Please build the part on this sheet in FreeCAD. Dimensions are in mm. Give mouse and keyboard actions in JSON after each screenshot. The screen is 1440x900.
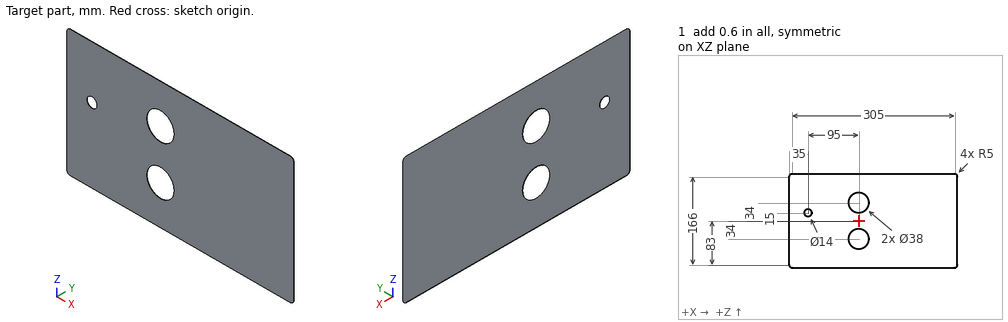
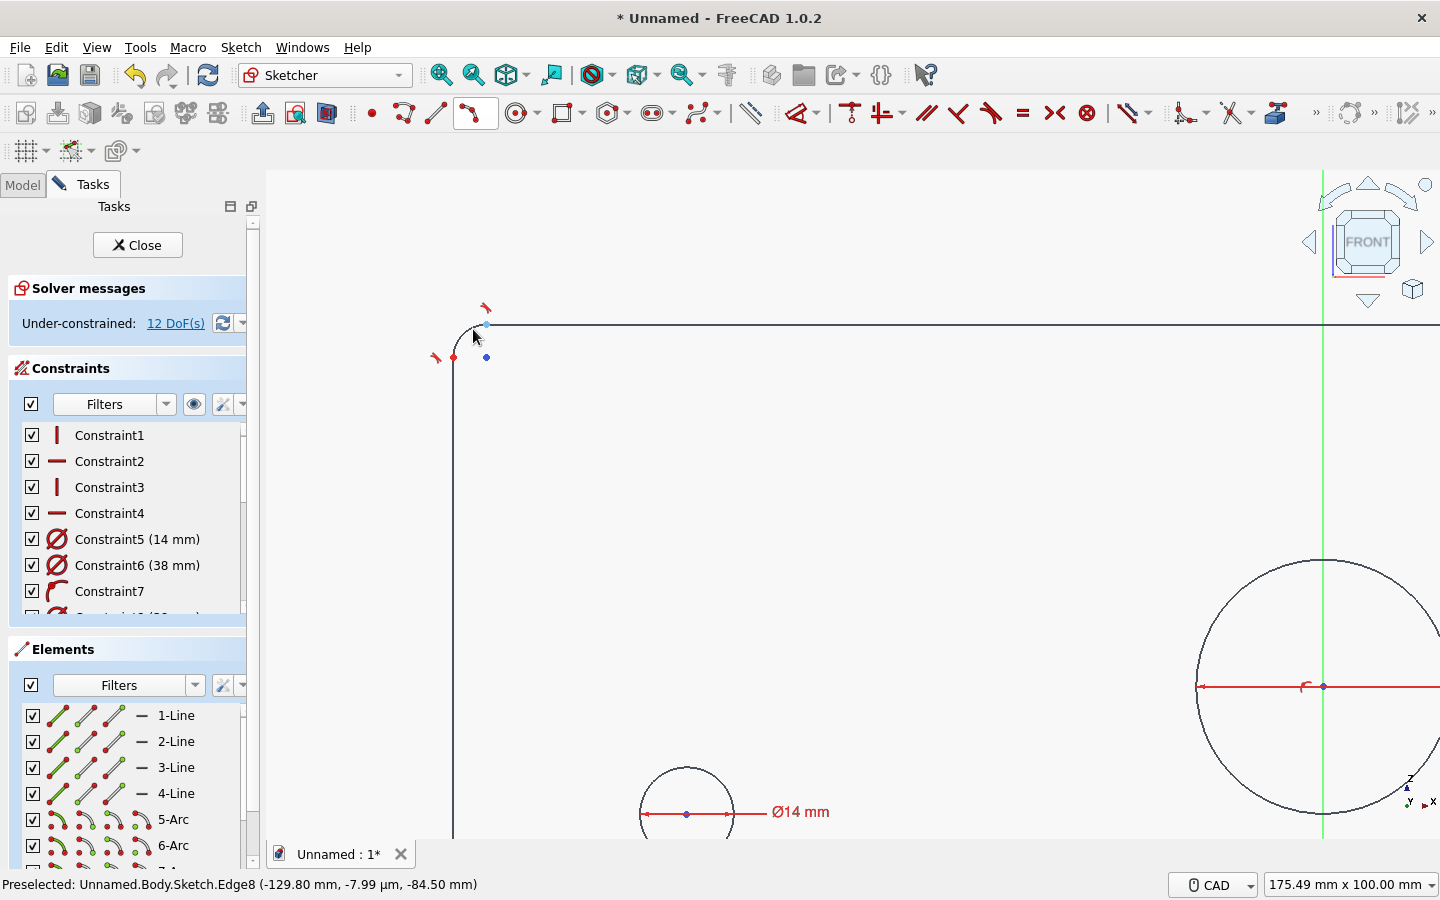
{"action": "left_click", "coordinate": [471, 328]}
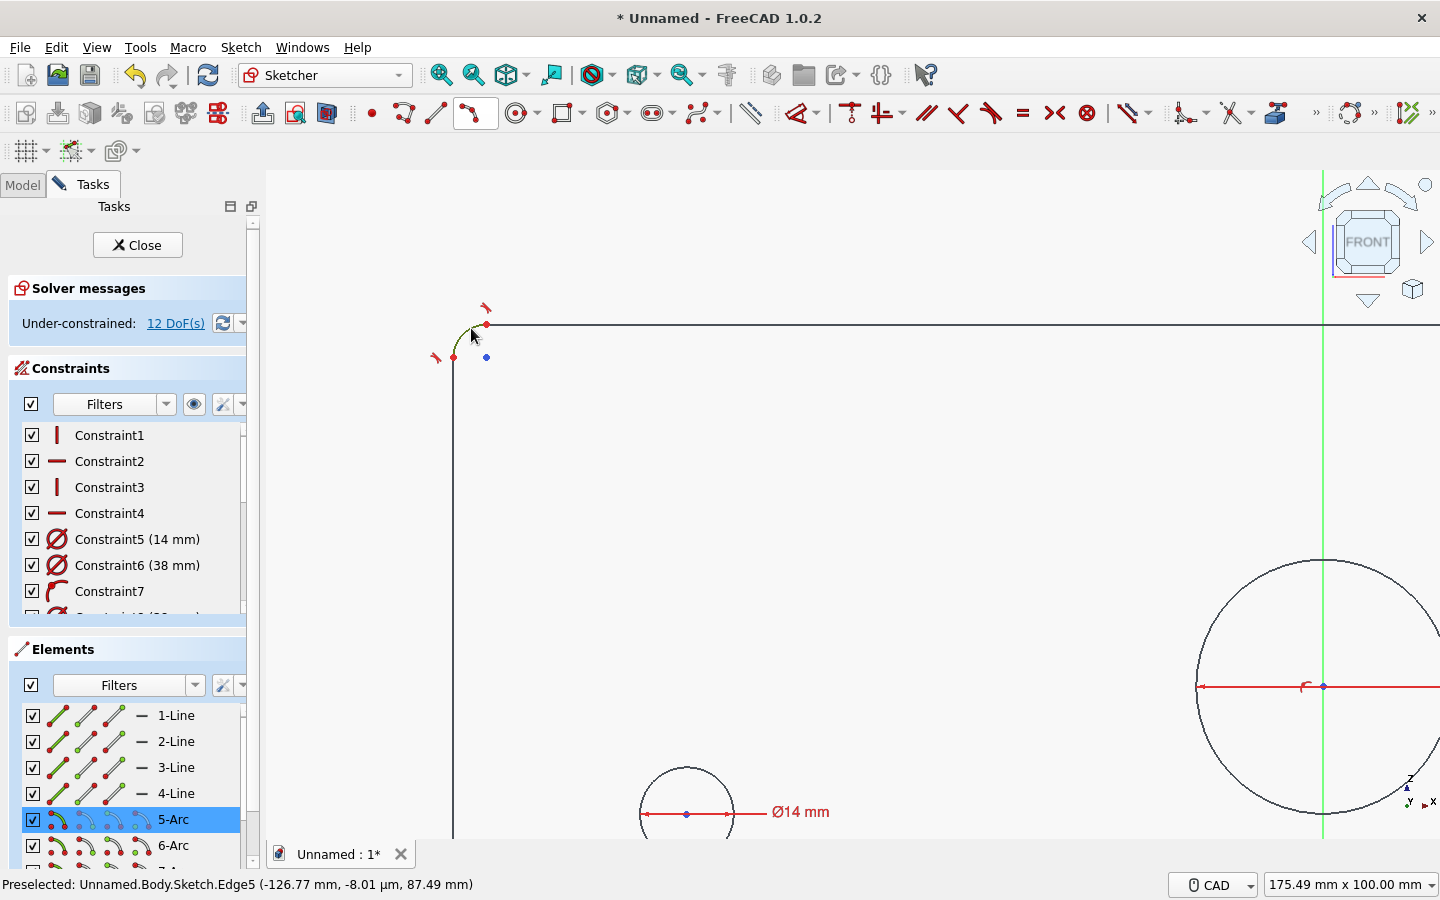
{"action": "scroll", "coordinate": [473, 329], "scroll_direction": "down", "scroll_amount": 6}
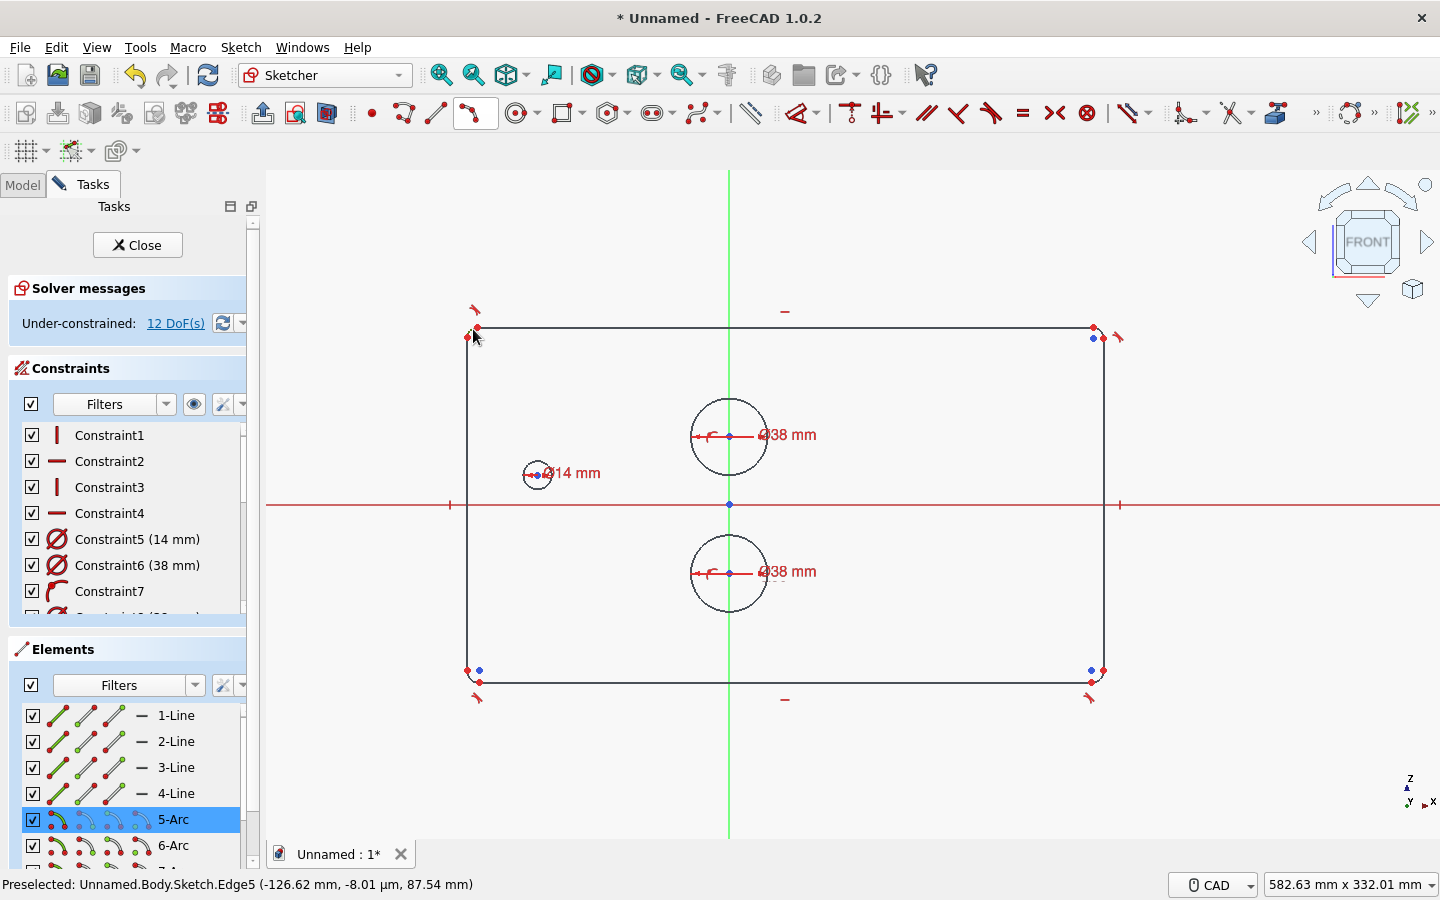
{"action": "scroll", "coordinate": [1102, 334], "scroll_direction": "up", "scroll_amount": 6}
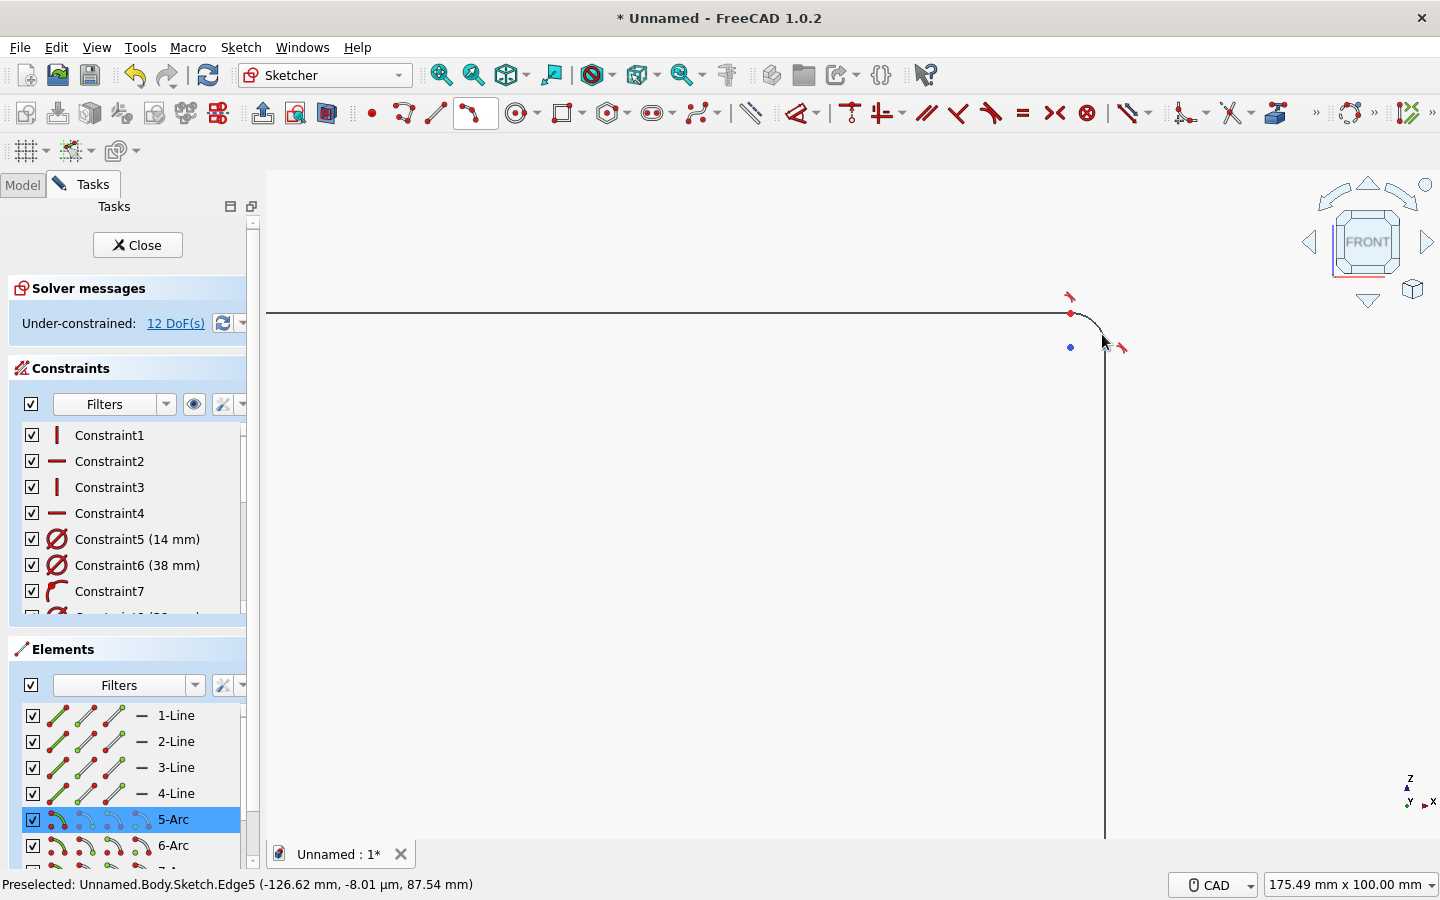
{"action": "left_click", "coordinate": [1102, 332]}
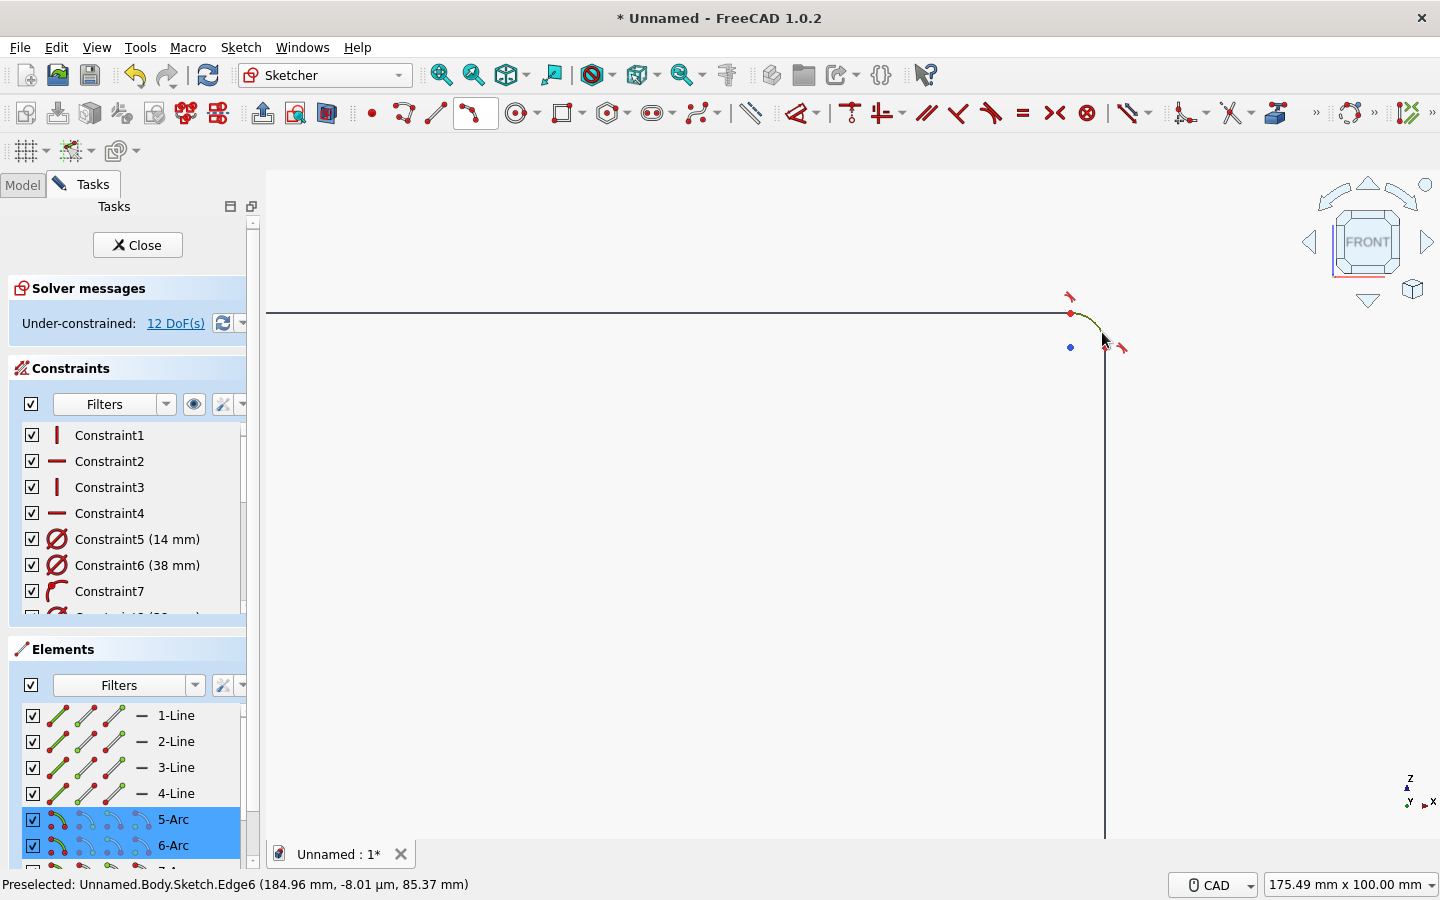
{"action": "scroll", "coordinate": [1103, 334], "scroll_direction": "down", "scroll_amount": 6}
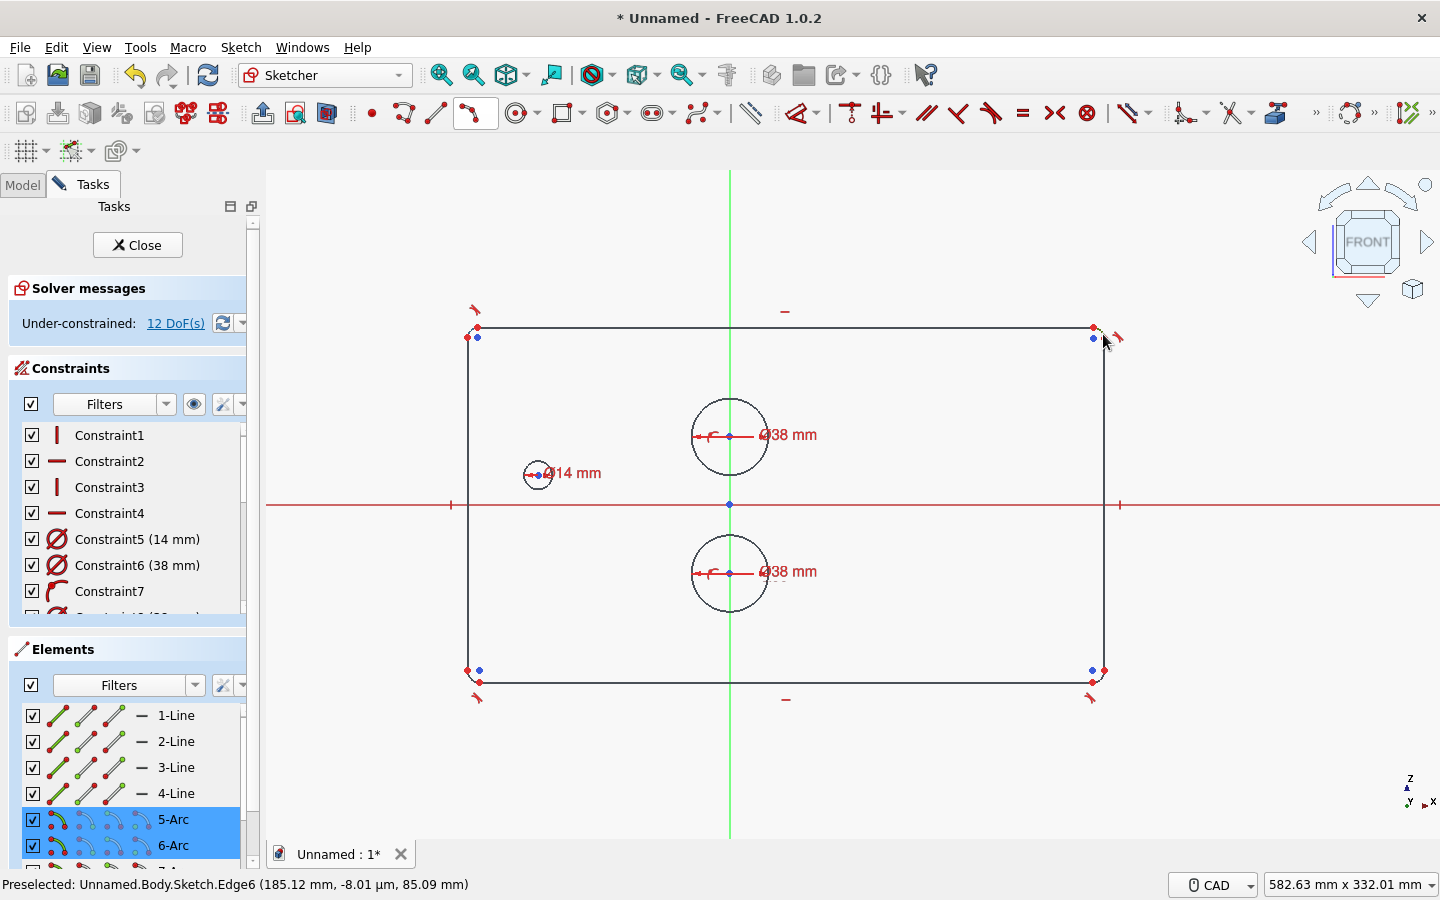
{"action": "scroll", "coordinate": [1098, 682], "scroll_direction": "up", "scroll_amount": 5}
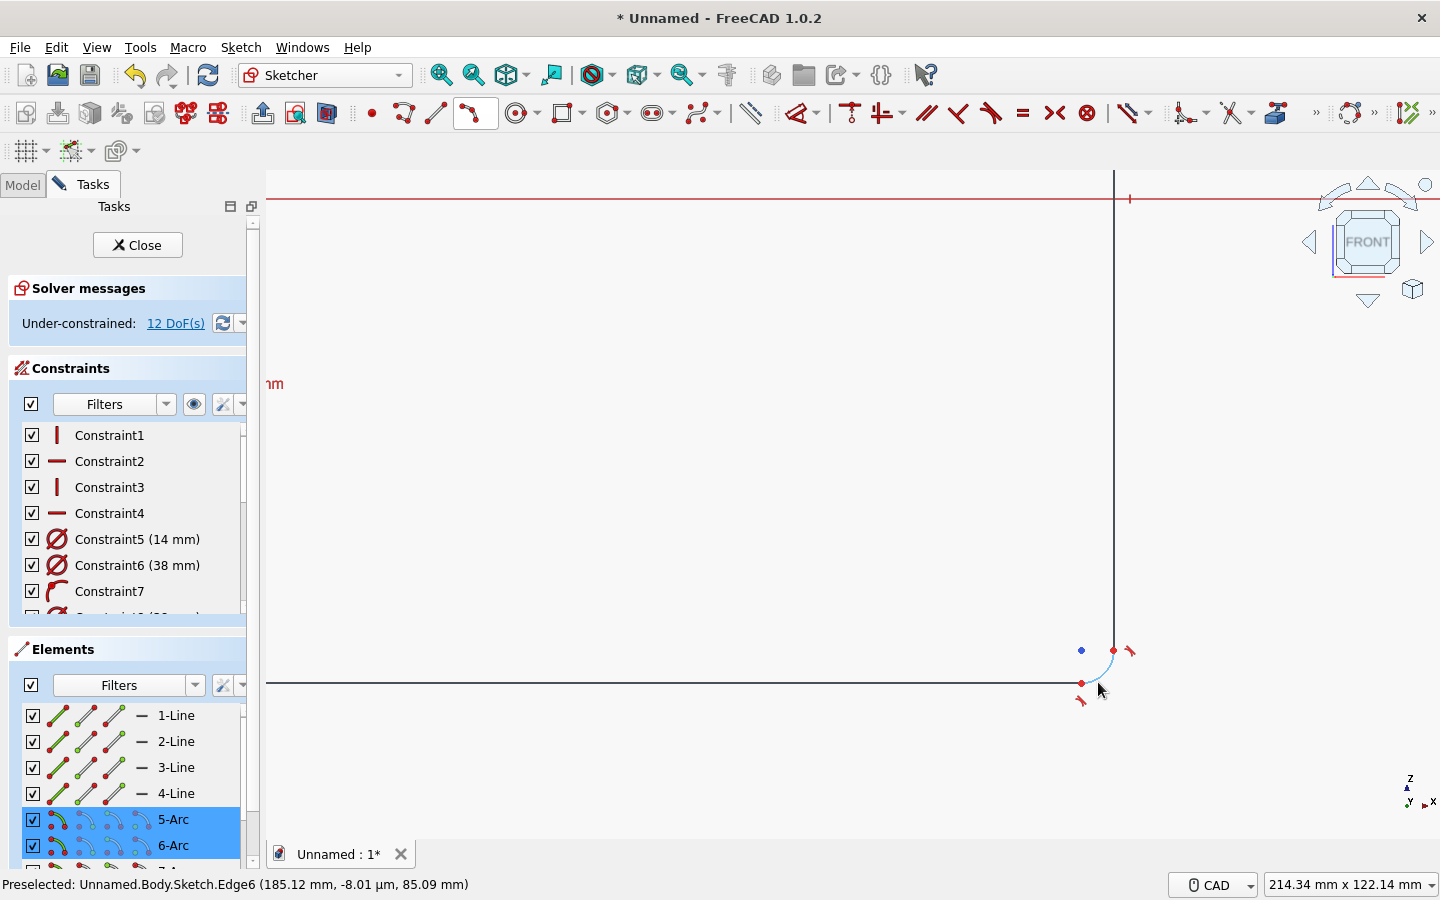
{"action": "left_click", "coordinate": [1096, 680]}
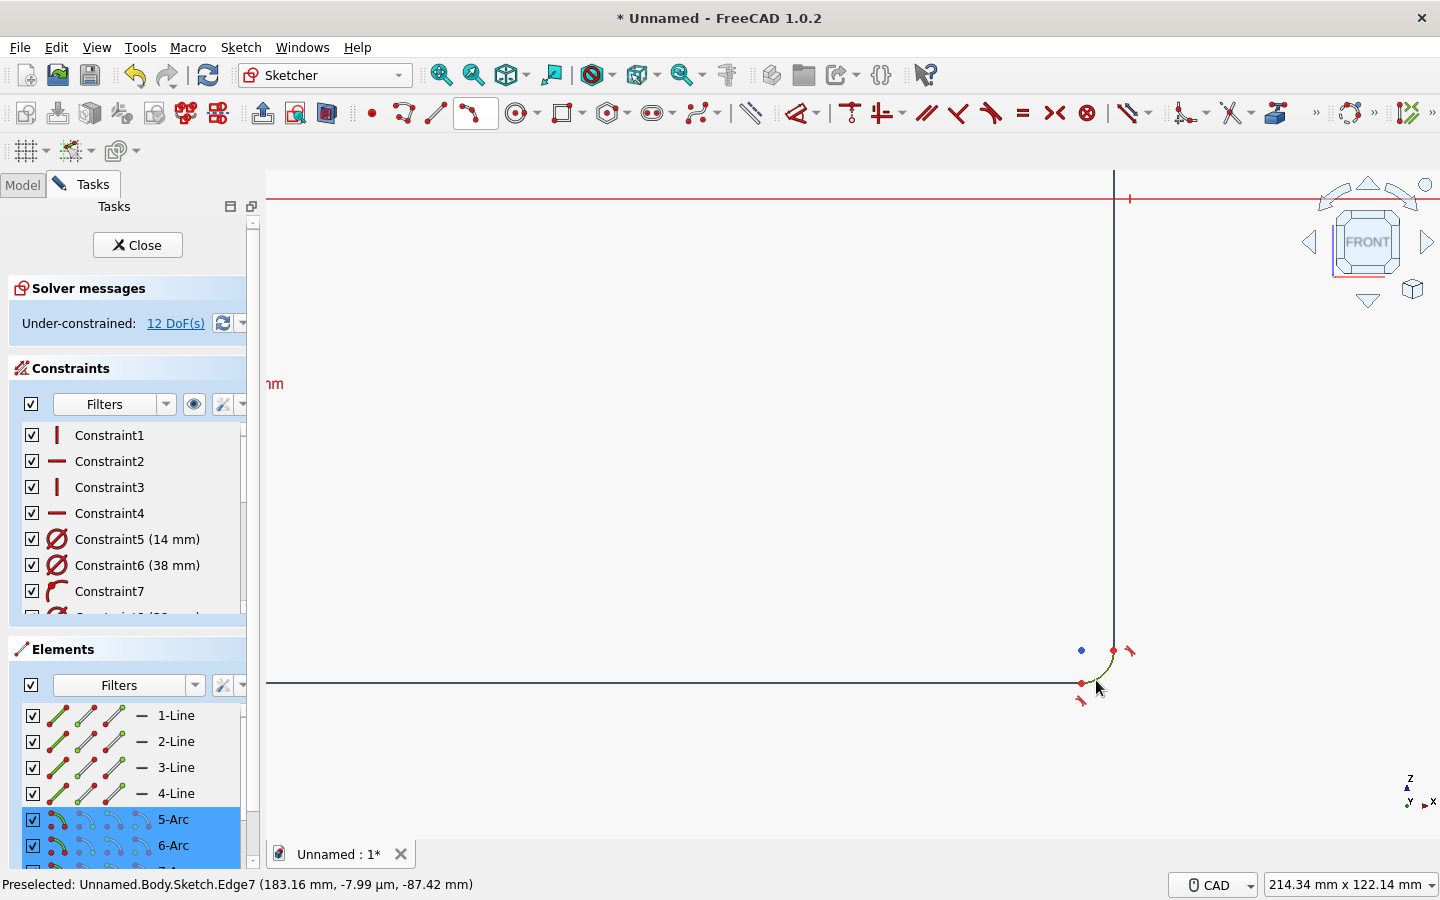
{"action": "scroll", "coordinate": [1097, 682], "scroll_direction": "down", "scroll_amount": 5}